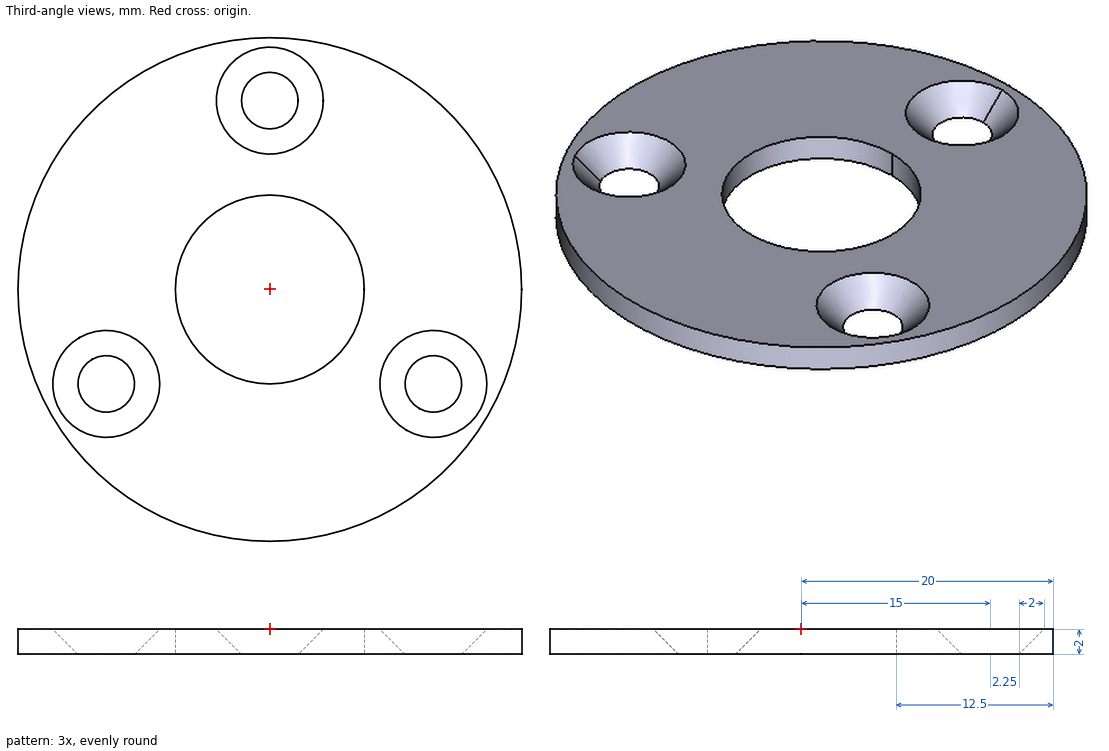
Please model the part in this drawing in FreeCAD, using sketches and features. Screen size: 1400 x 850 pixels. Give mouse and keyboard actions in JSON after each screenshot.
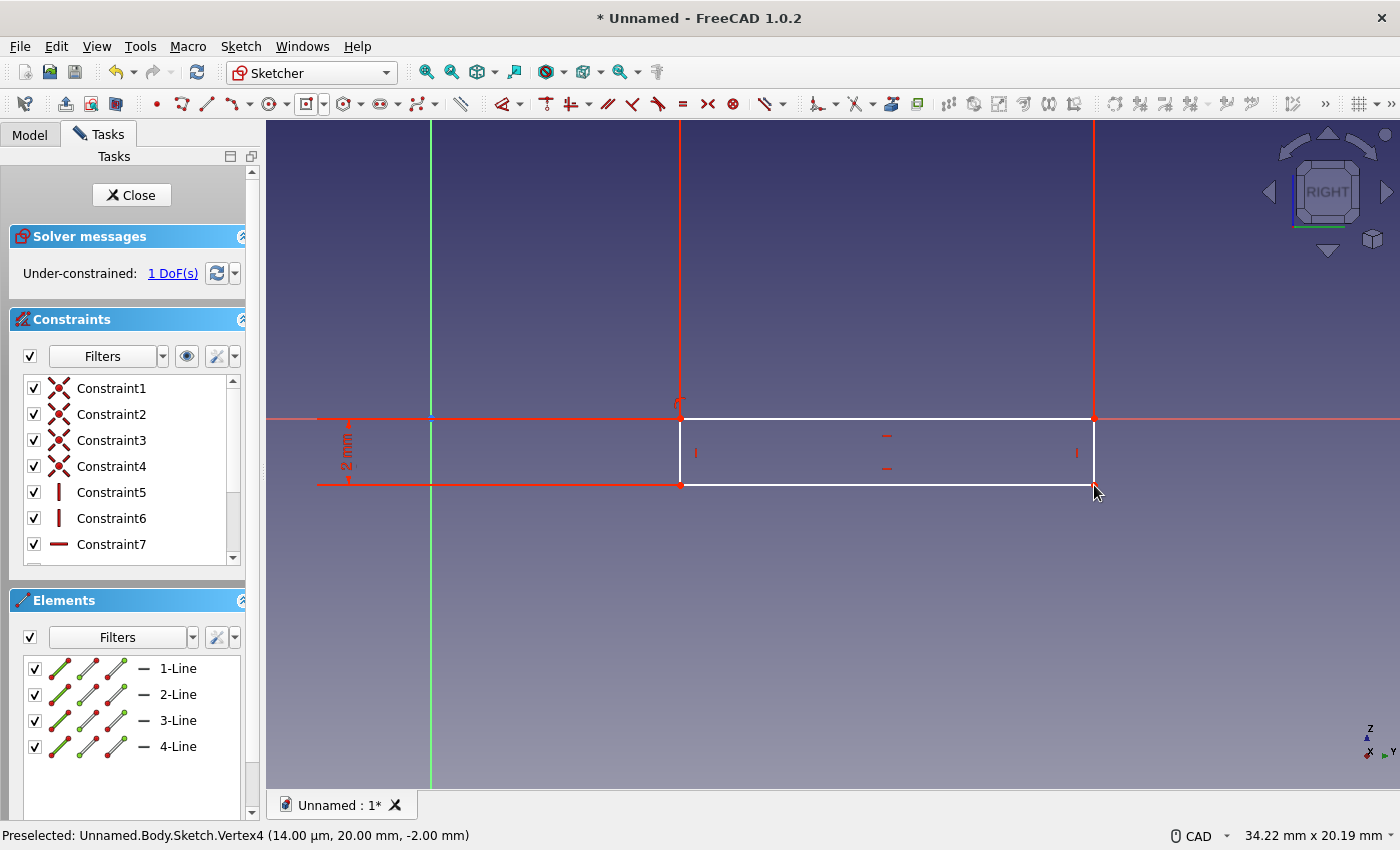
{"action": "left_click", "coordinate": [502, 104]}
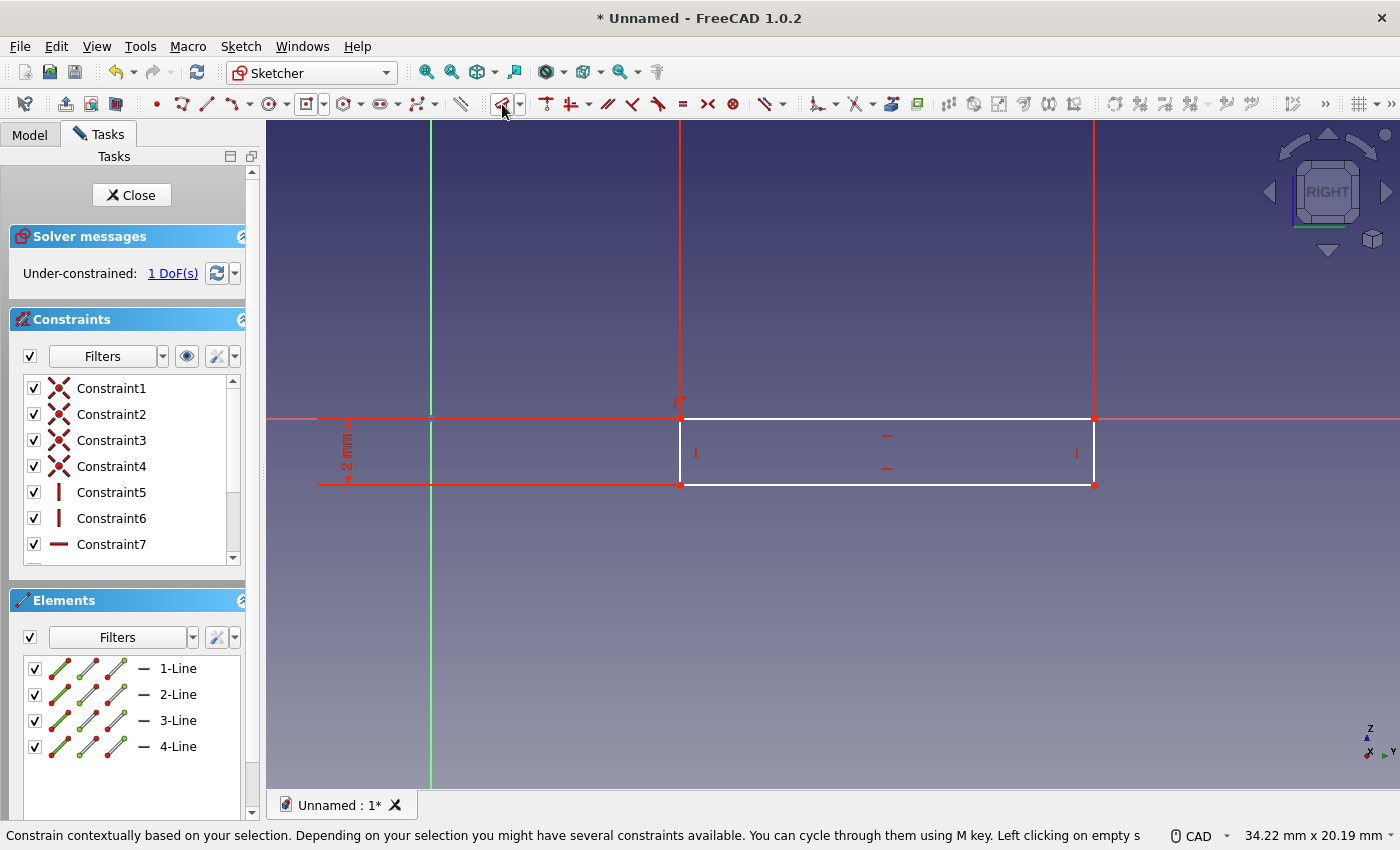
{"action": "left_click", "coordinate": [1094, 485]}
{"action": "left_click", "coordinate": [763, 519]}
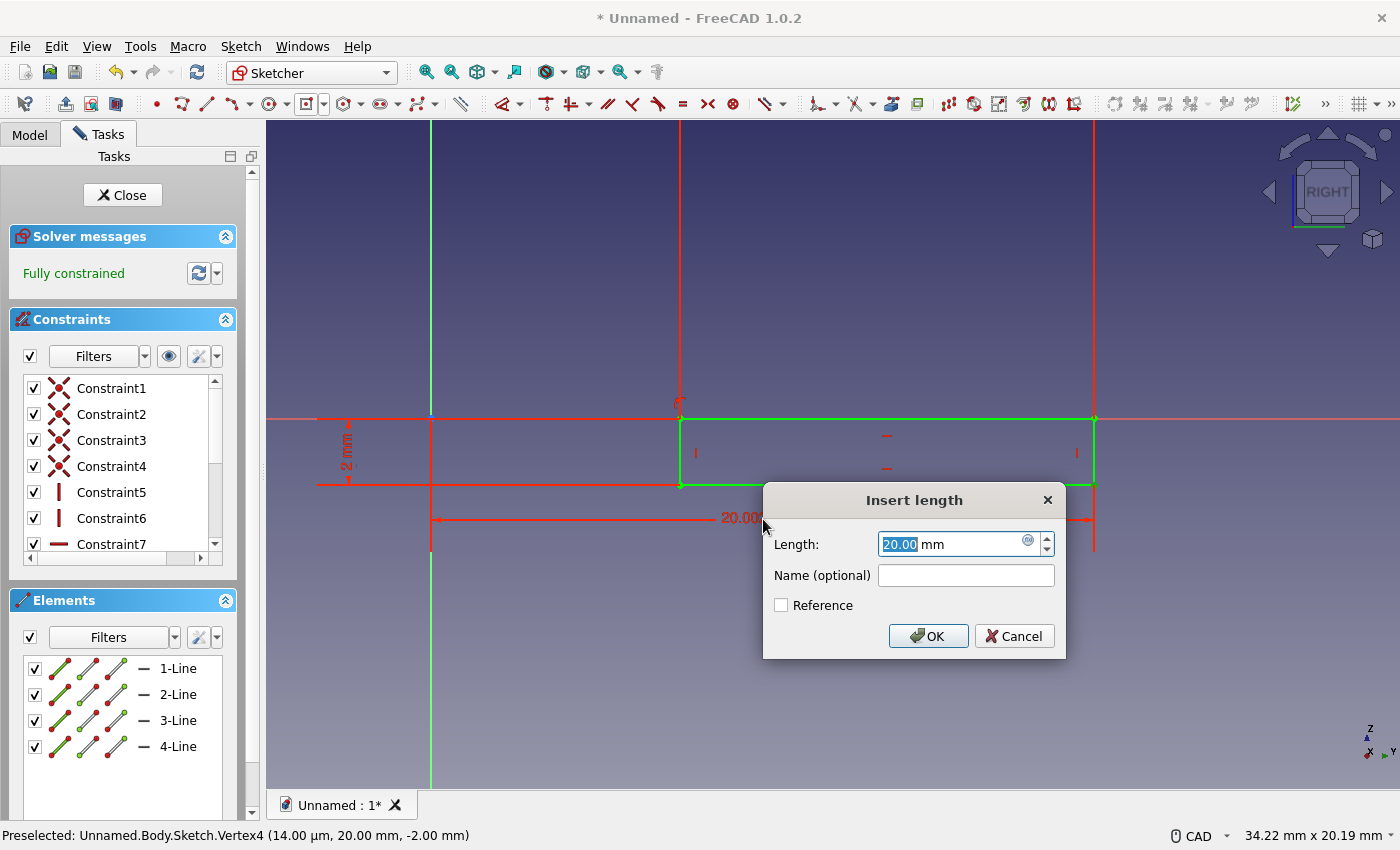
{"action": "type", "text": "20"}
{"action": "key", "text": "Return"}
{"action": "key", "text": "Escape"}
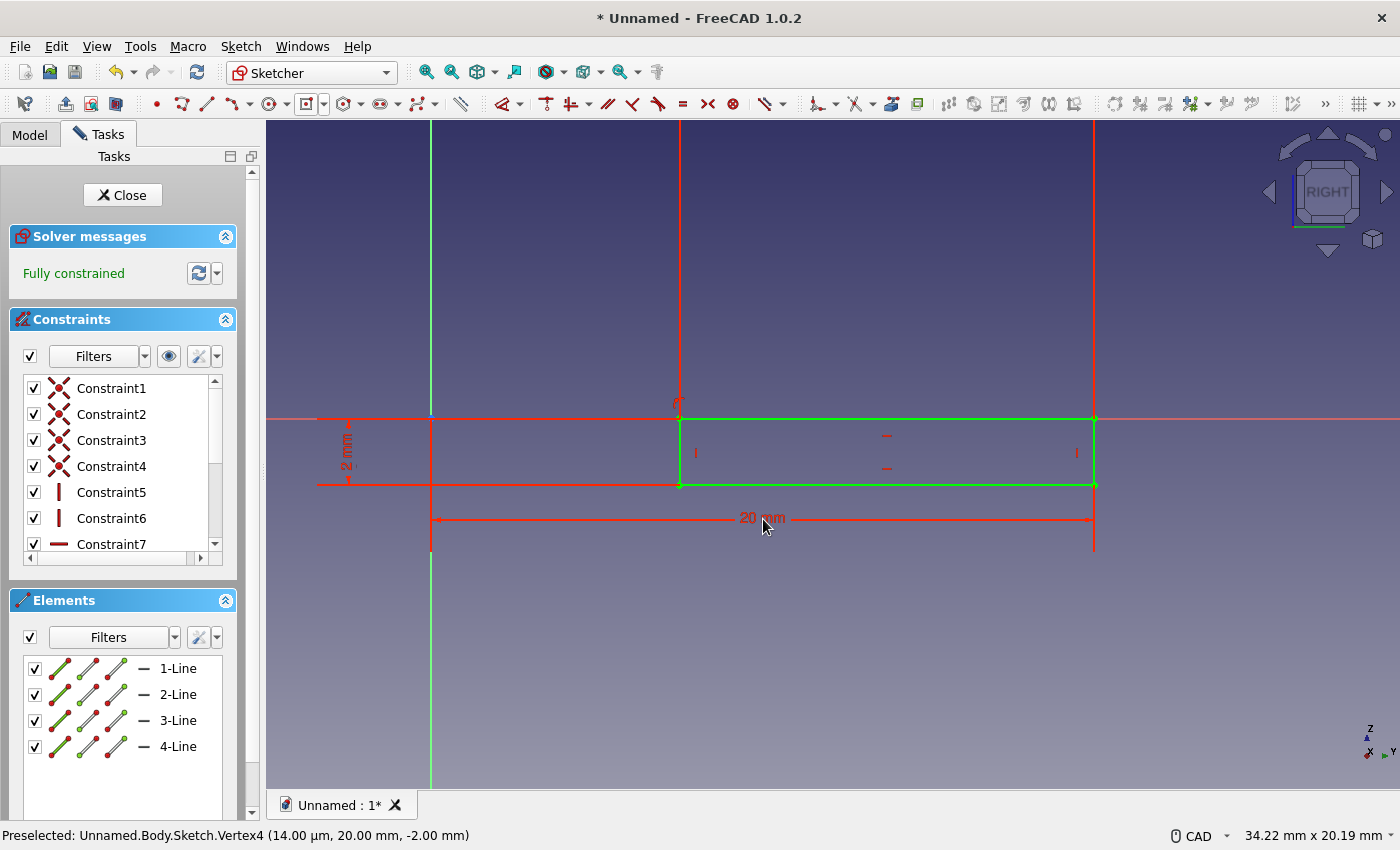
{"action": "left_click", "coordinate": [123, 195]}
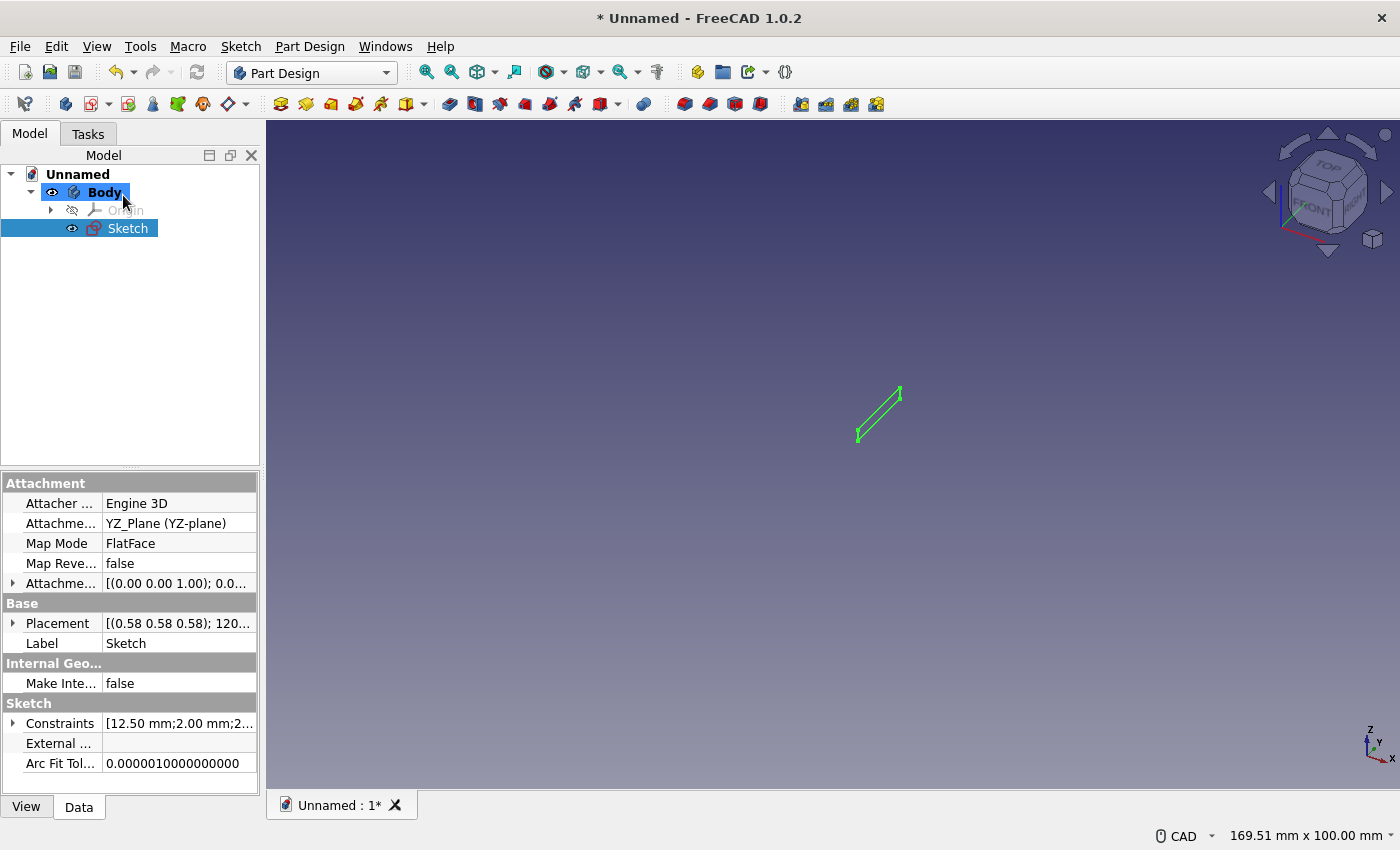
{"action": "left_click", "coordinate": [306, 104]}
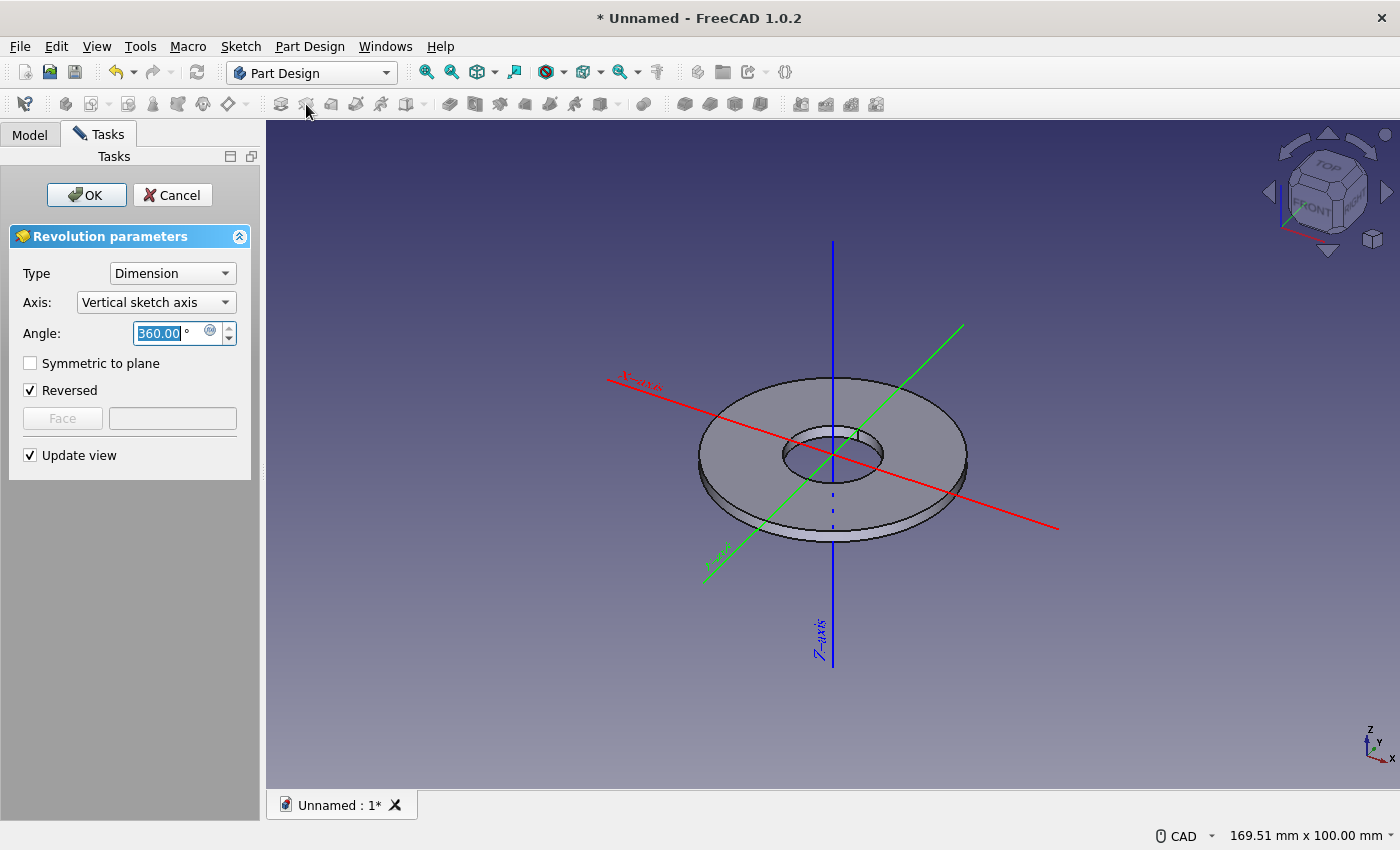
{"action": "left_click", "coordinate": [87, 195]}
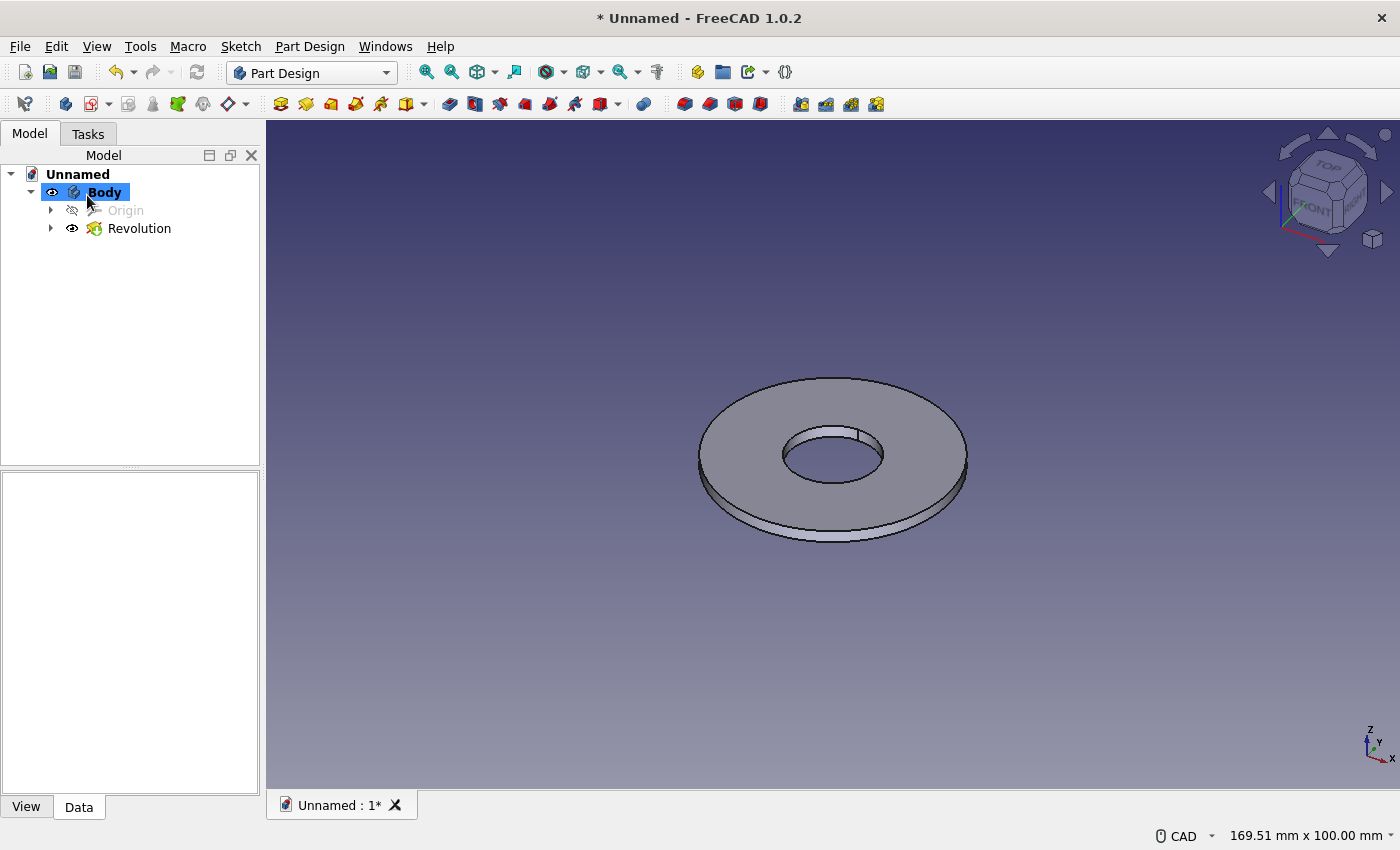
{"action": "left_click", "coordinate": [427, 72]}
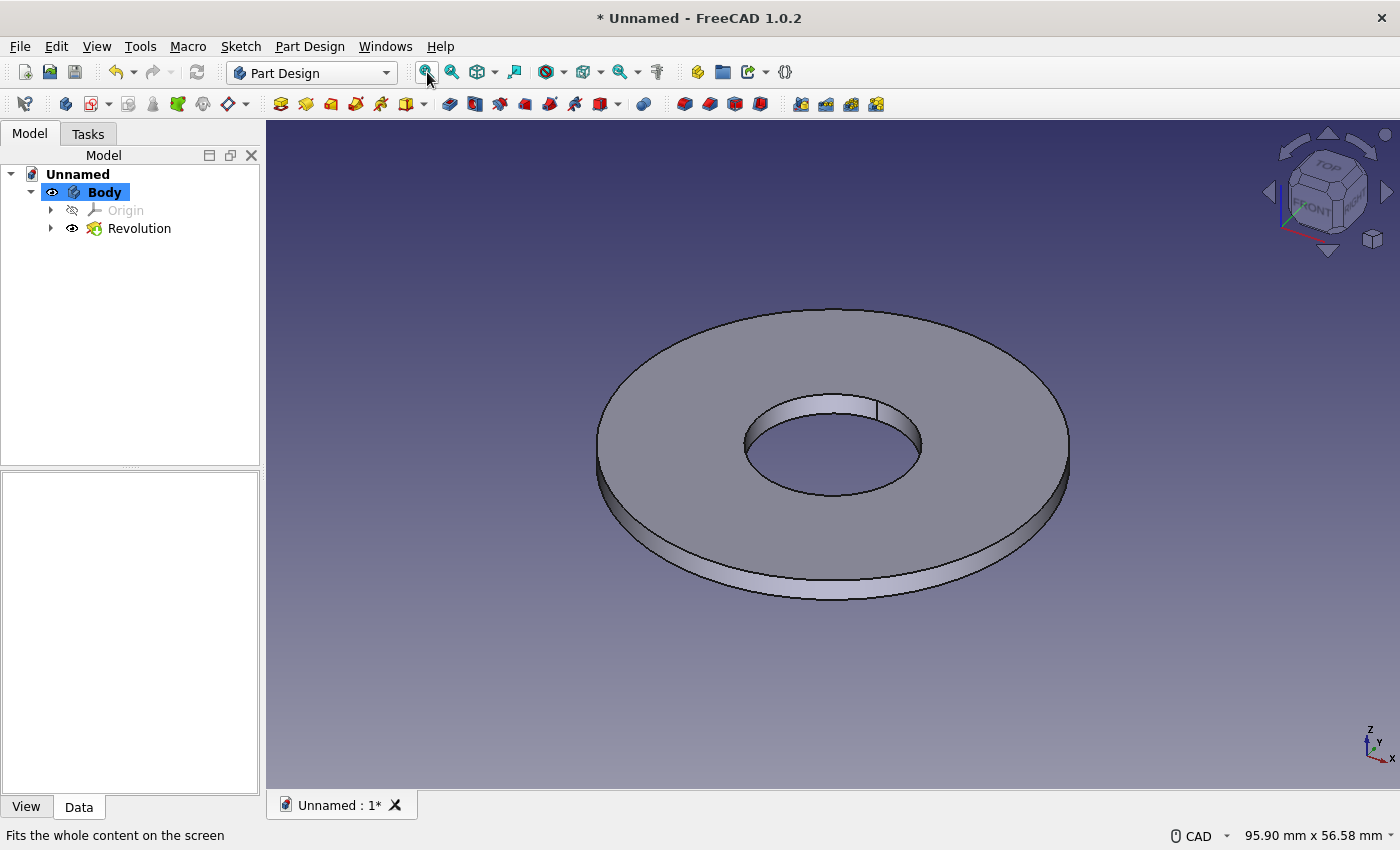
{"action": "left_click", "coordinate": [90, 104]}